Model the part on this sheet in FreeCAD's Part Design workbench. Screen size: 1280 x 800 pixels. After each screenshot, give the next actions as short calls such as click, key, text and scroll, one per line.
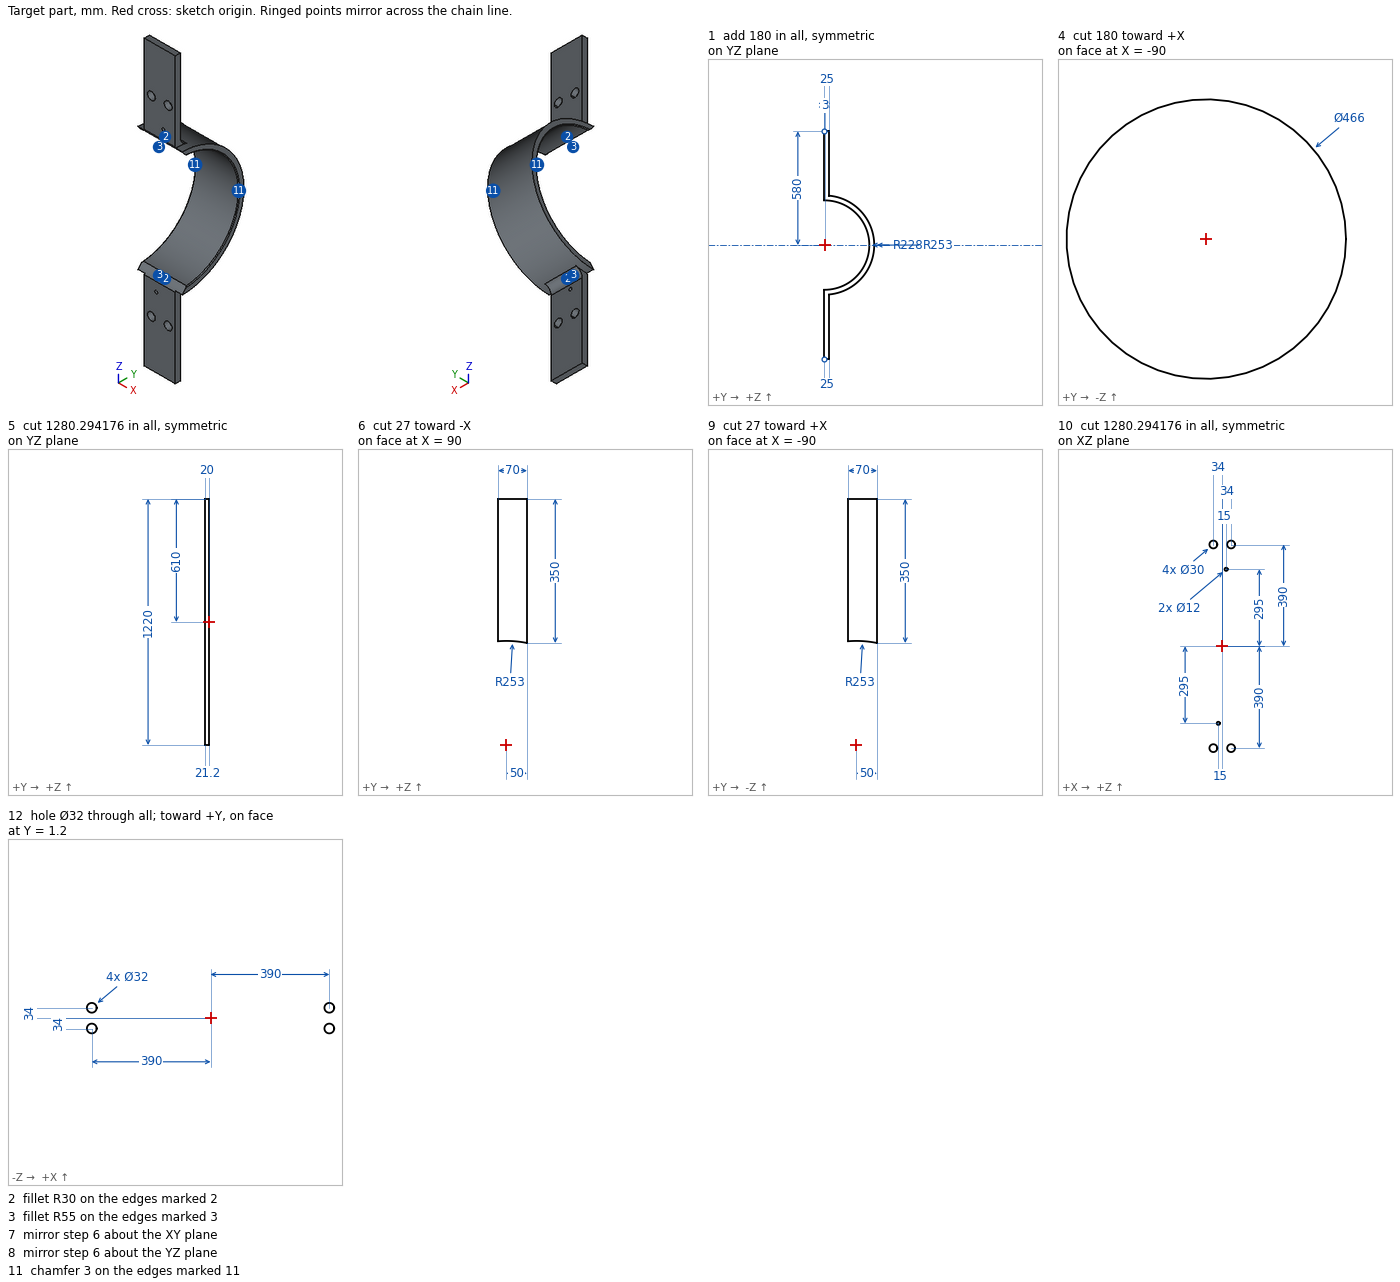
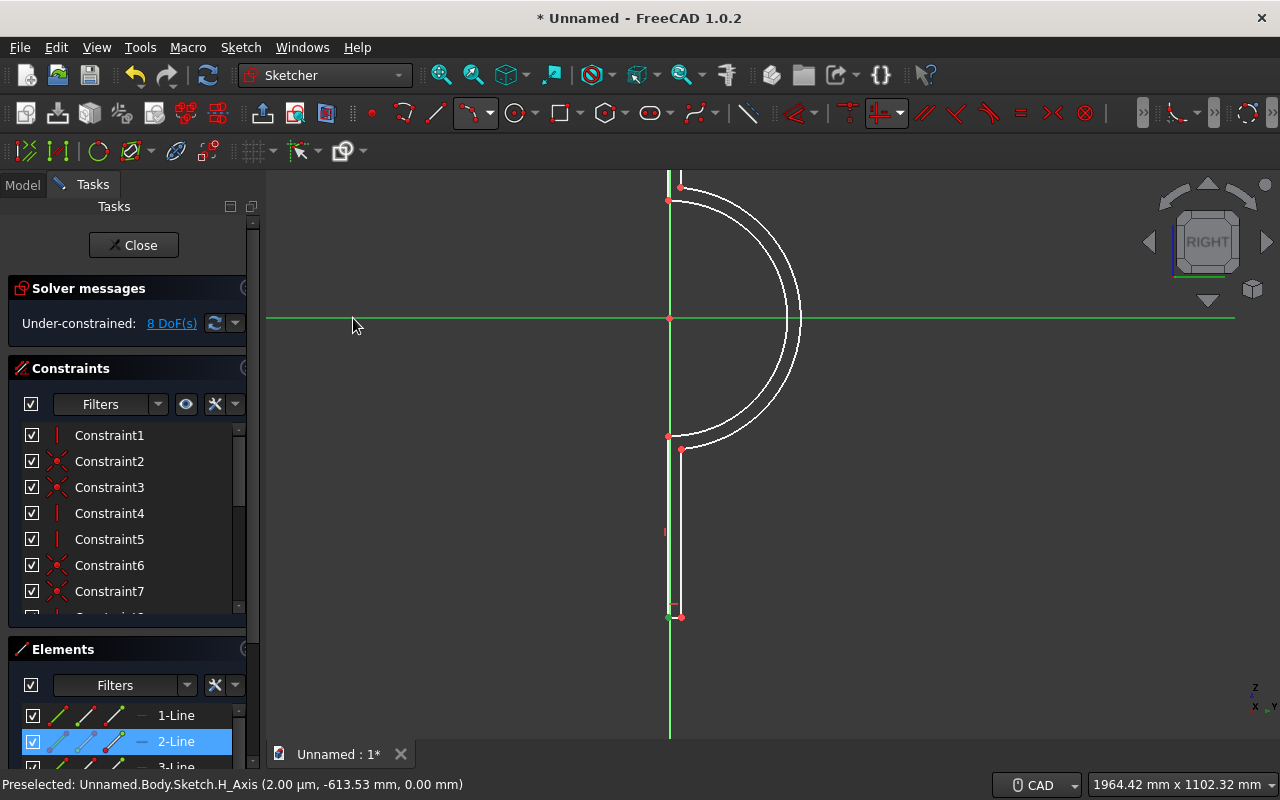
click(1054, 114)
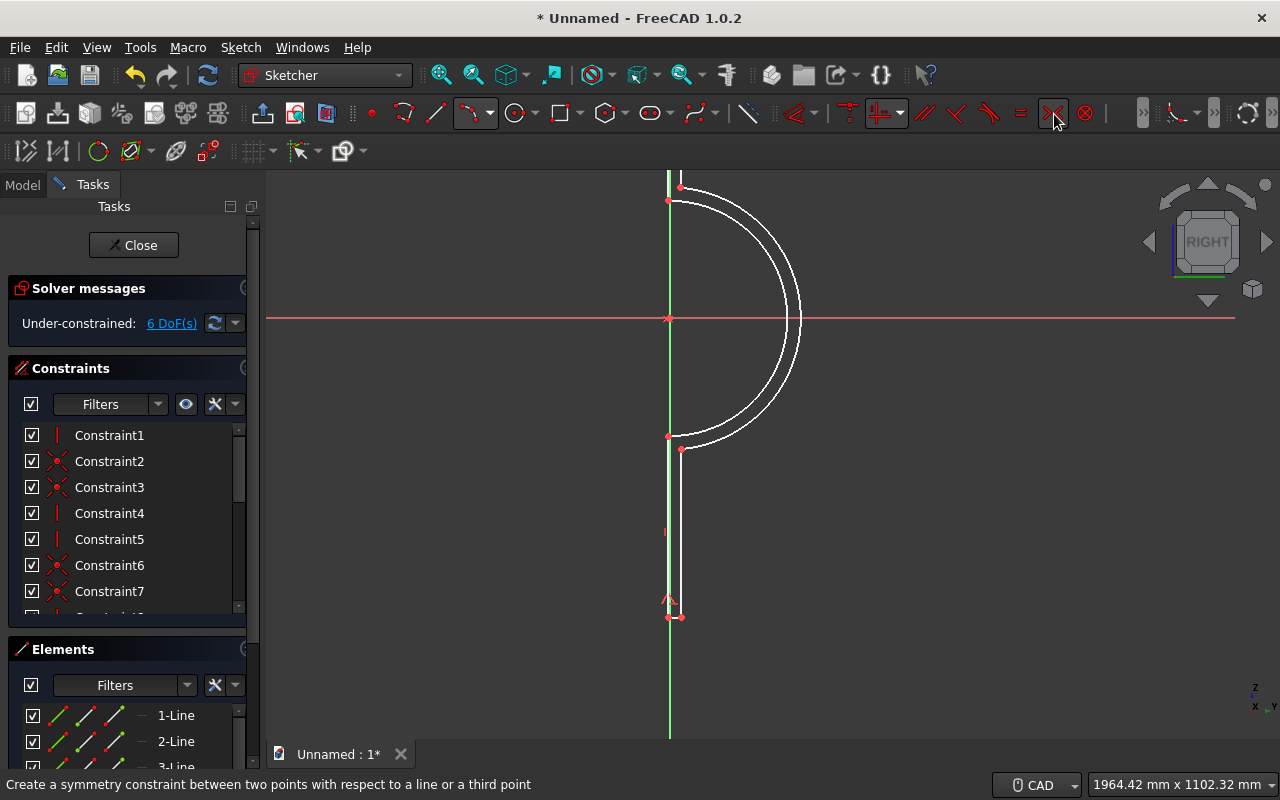
click(794, 114)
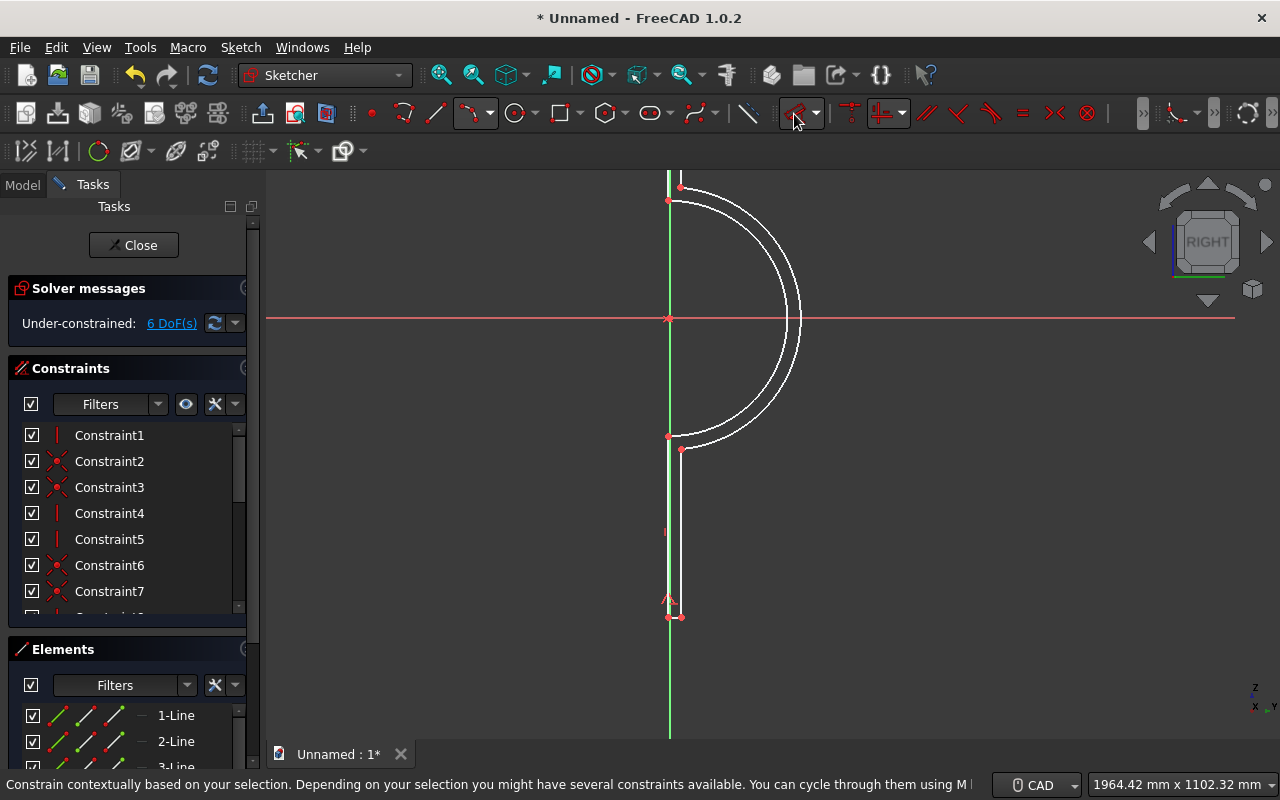
click(765, 388)
click(791, 407)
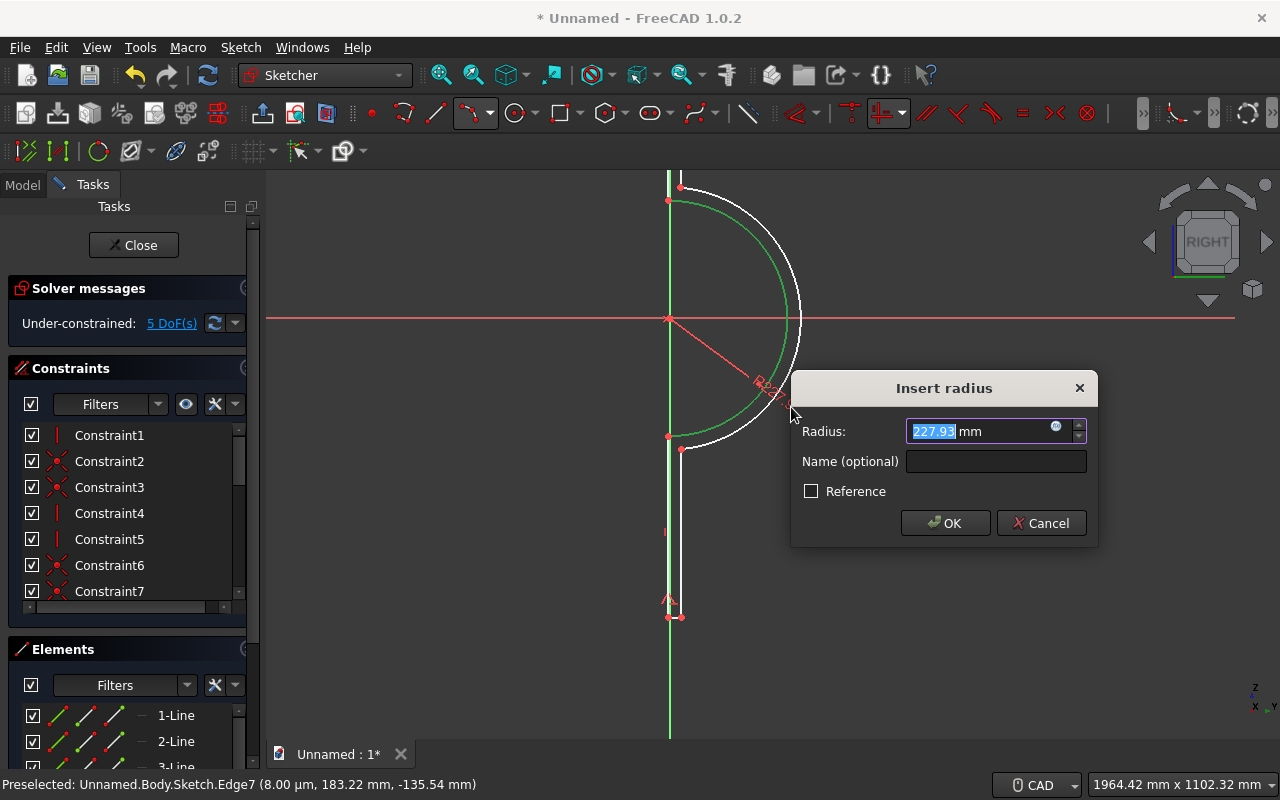
text(228)
key(Return)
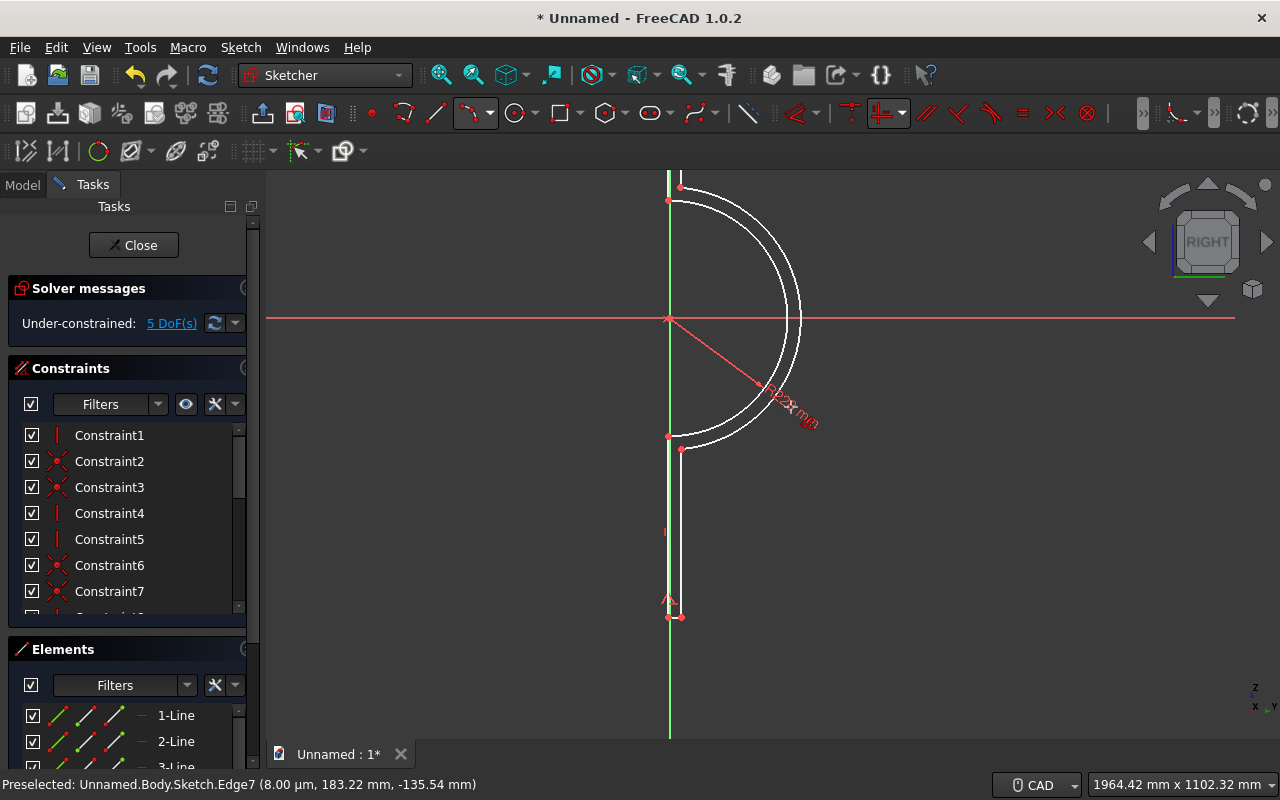
click(779, 392)
click(745, 464)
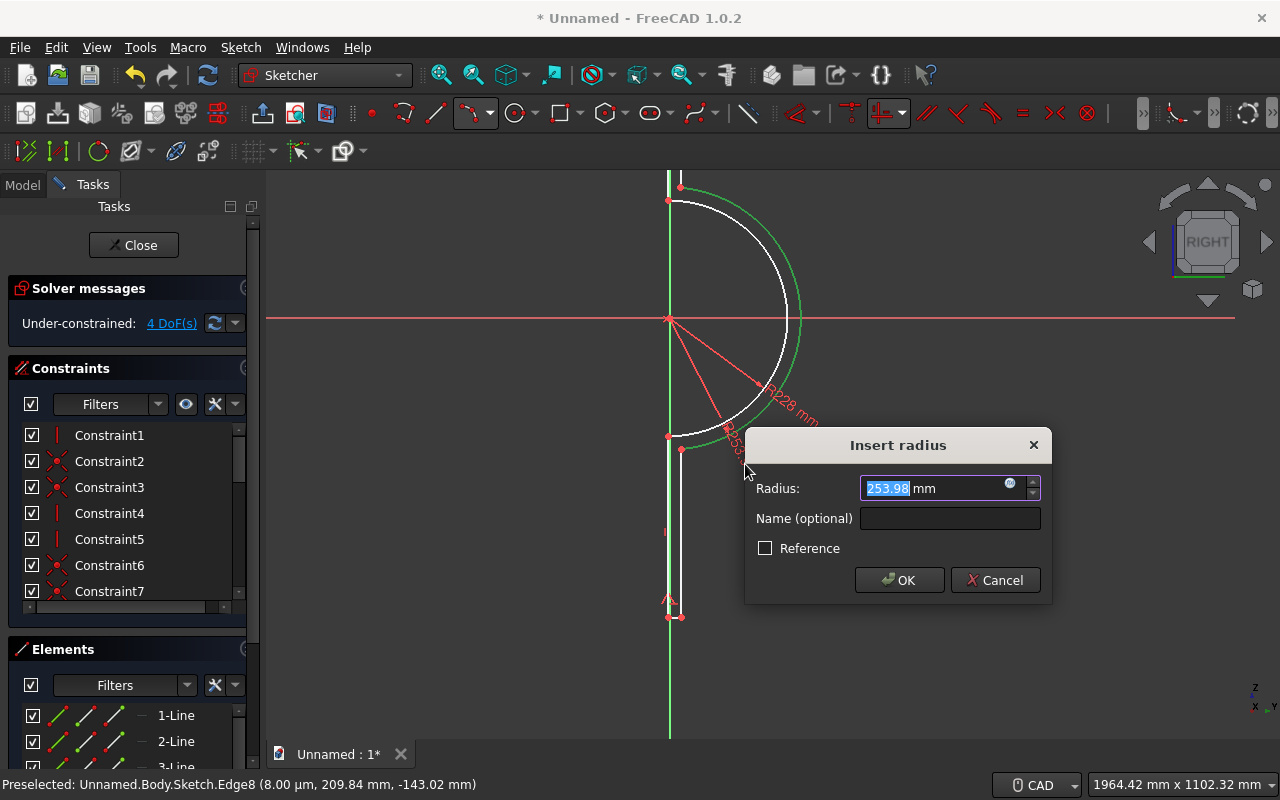
text(253)
key(Return)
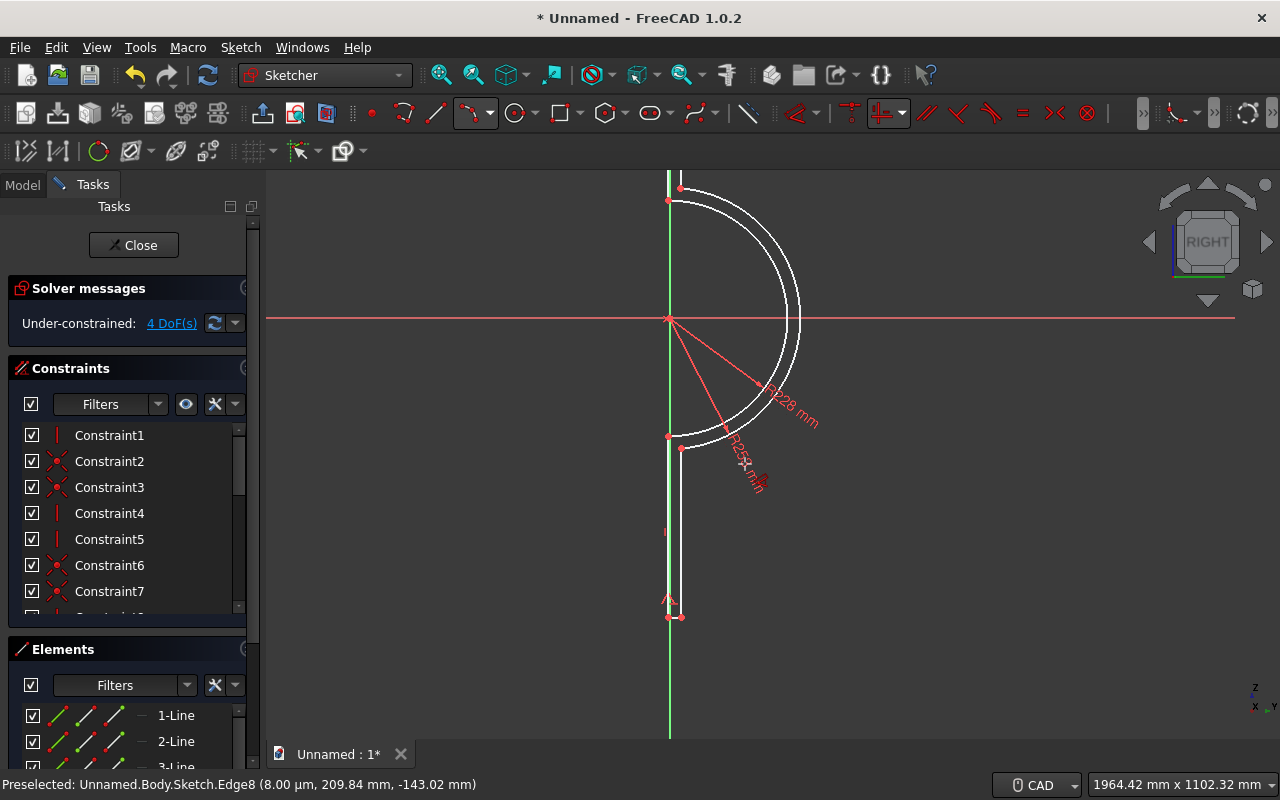
scroll(668, 620, down, 3)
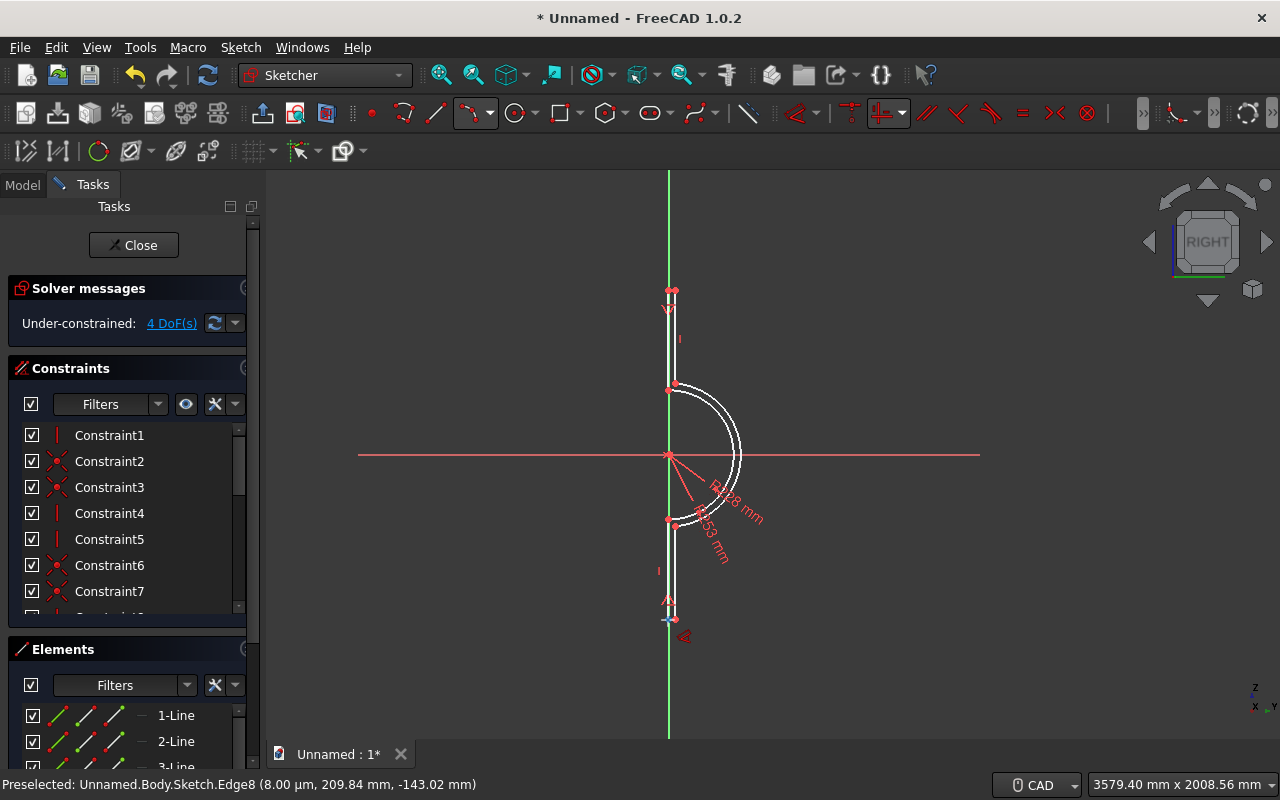
scroll(672, 291, up, 9)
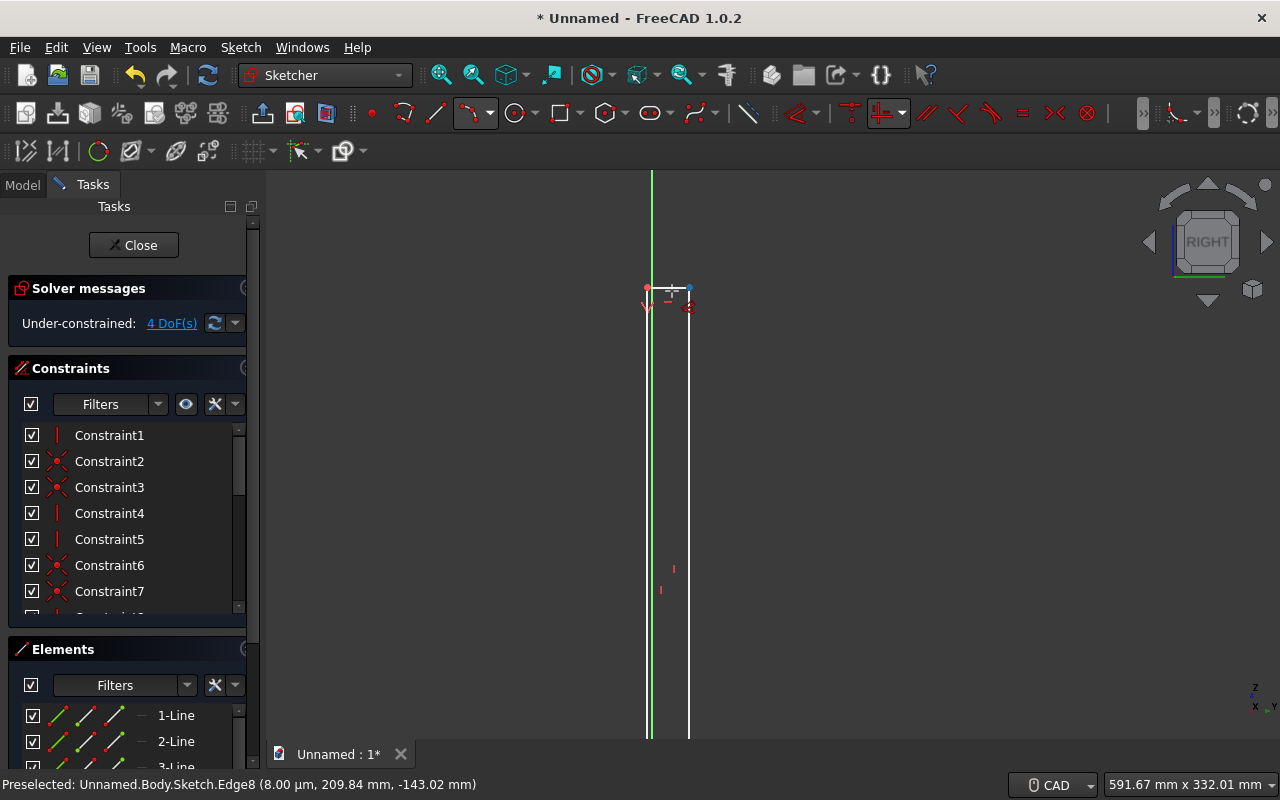
click(672, 288)
click(668, 254)